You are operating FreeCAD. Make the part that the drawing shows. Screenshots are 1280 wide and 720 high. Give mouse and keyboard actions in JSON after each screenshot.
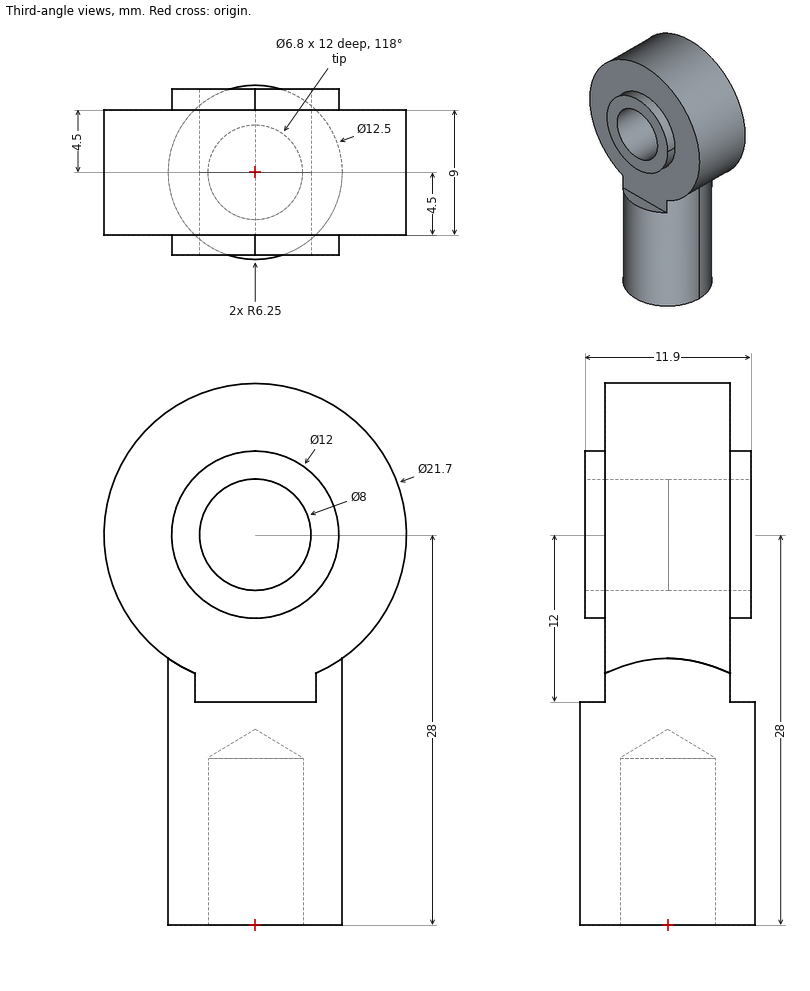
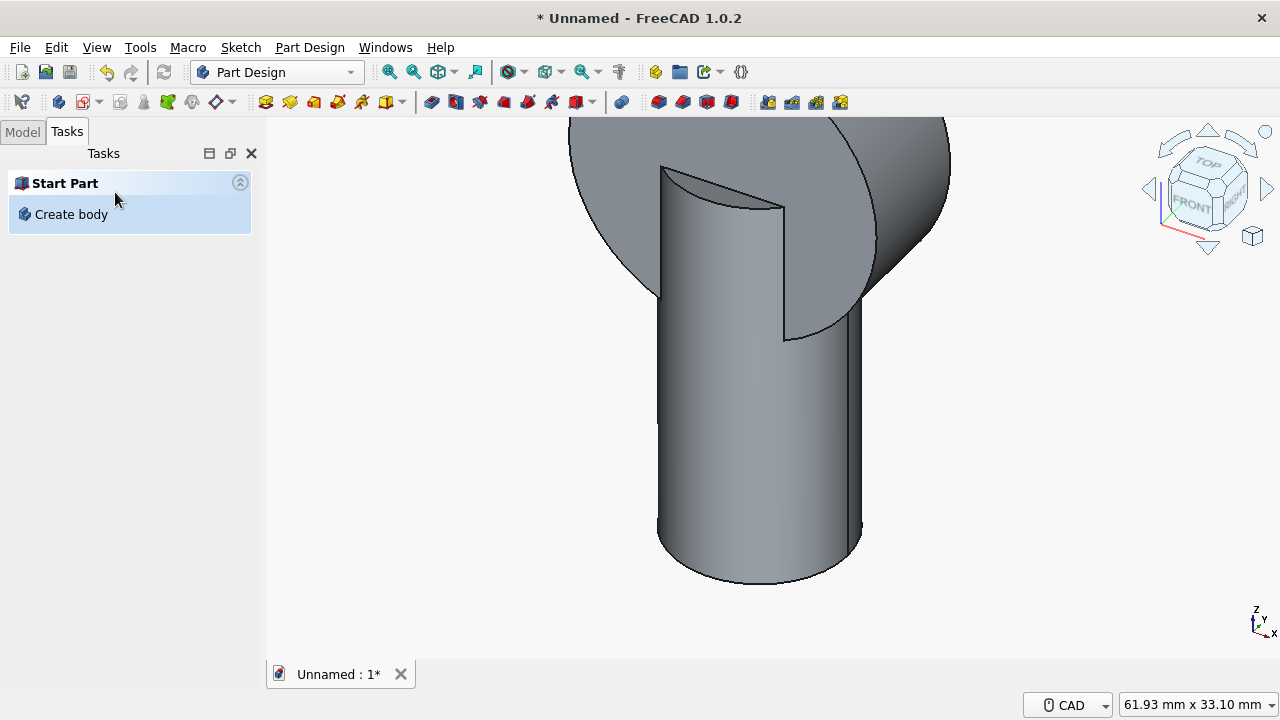
{"action": "key", "text": "v f"}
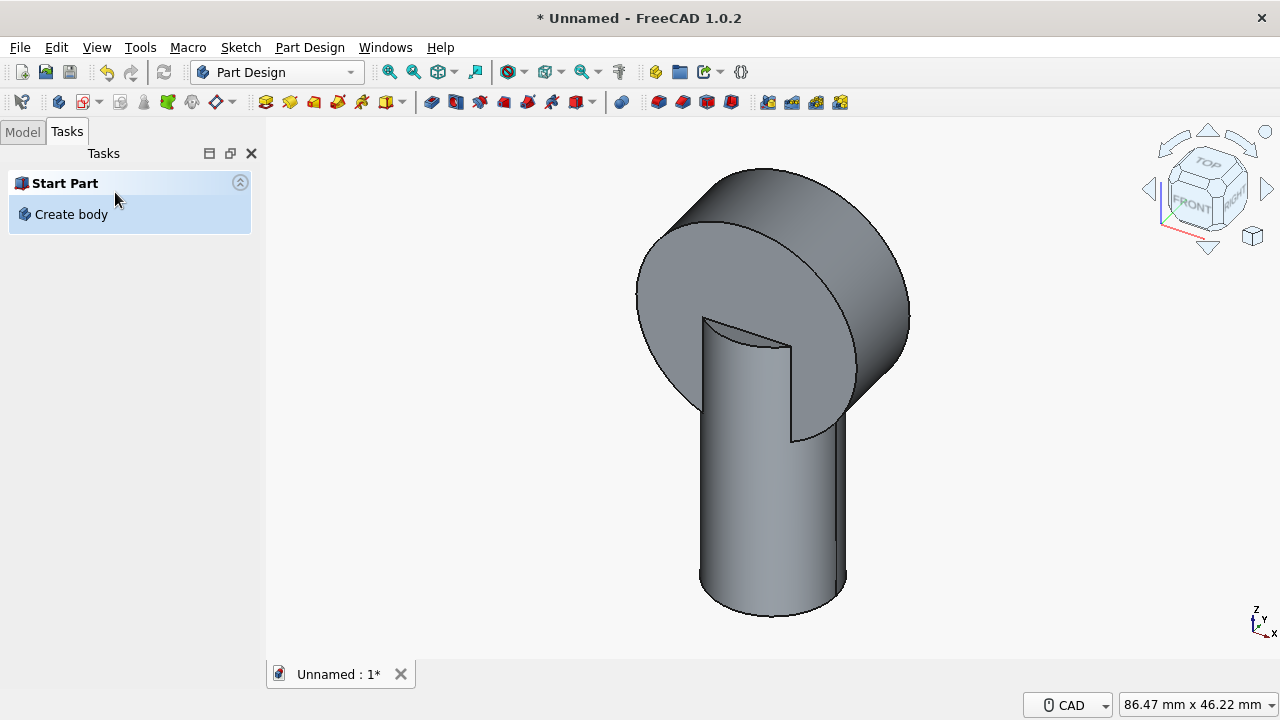
{"action": "left_click", "coordinate": [23, 131]}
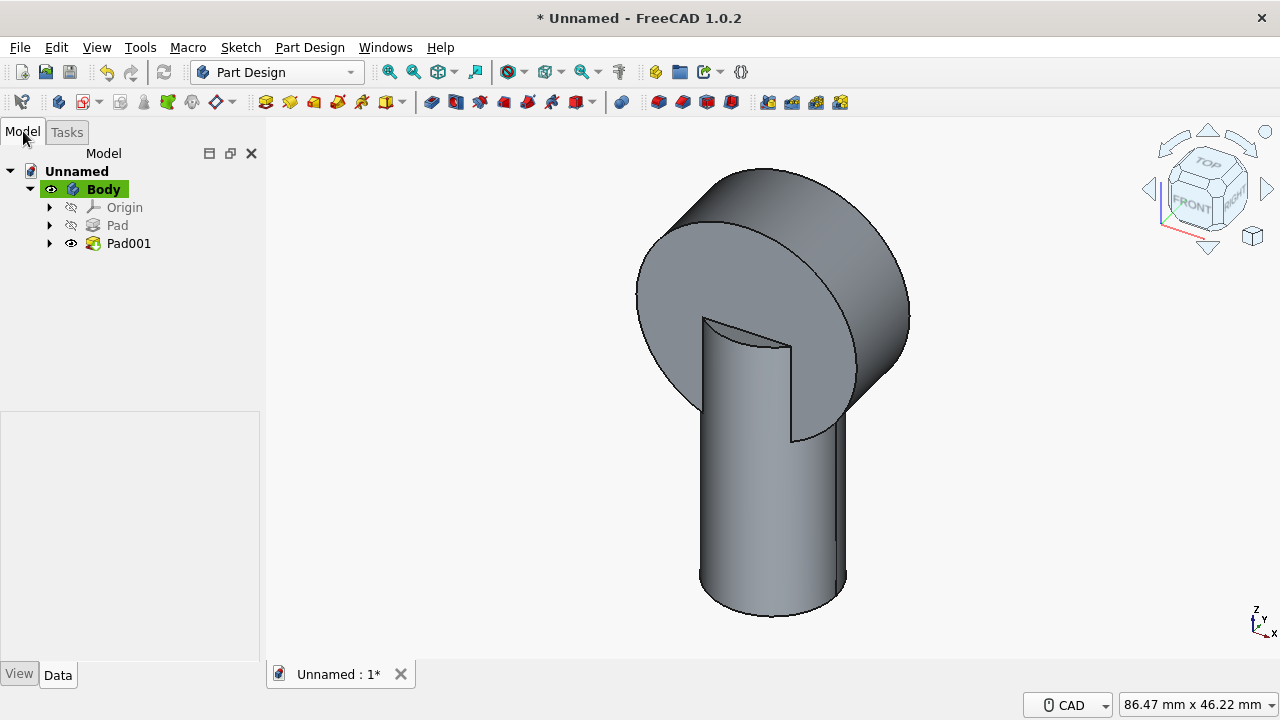
{"action": "left_click", "coordinate": [50, 207]}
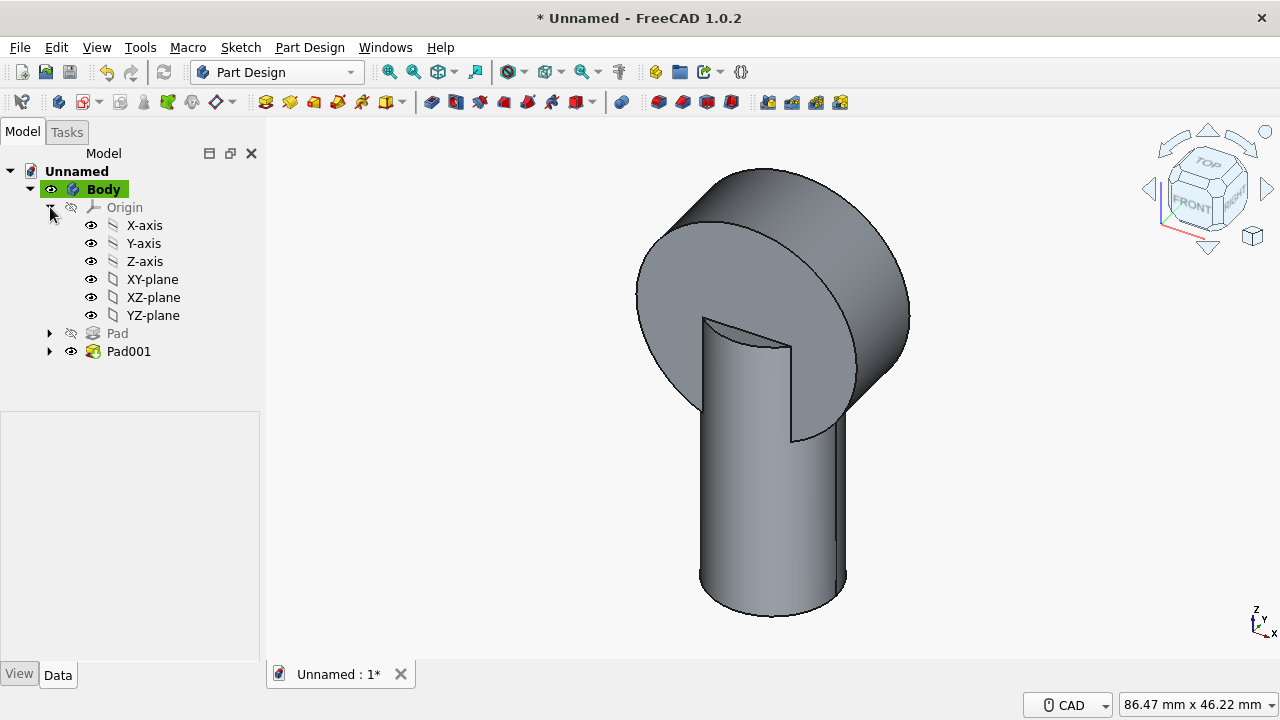
{"action": "left_click", "coordinate": [136, 279]}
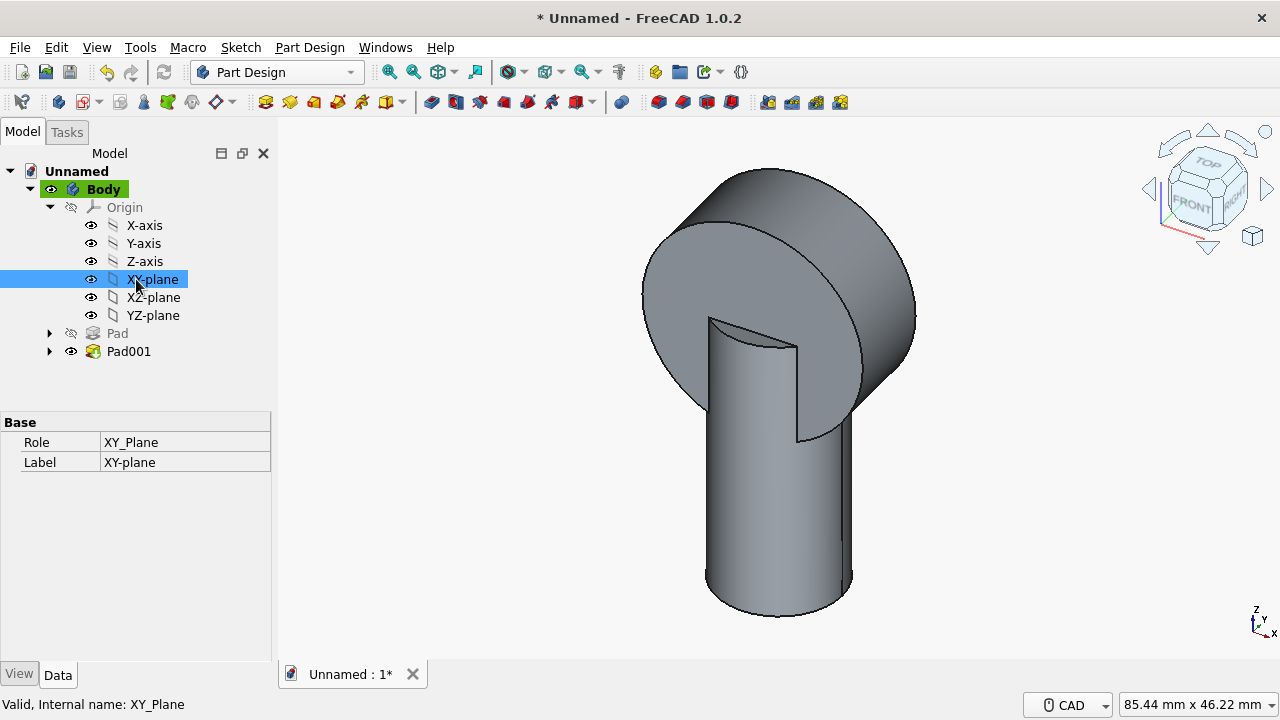
{"action": "left_click", "coordinate": [216, 102]}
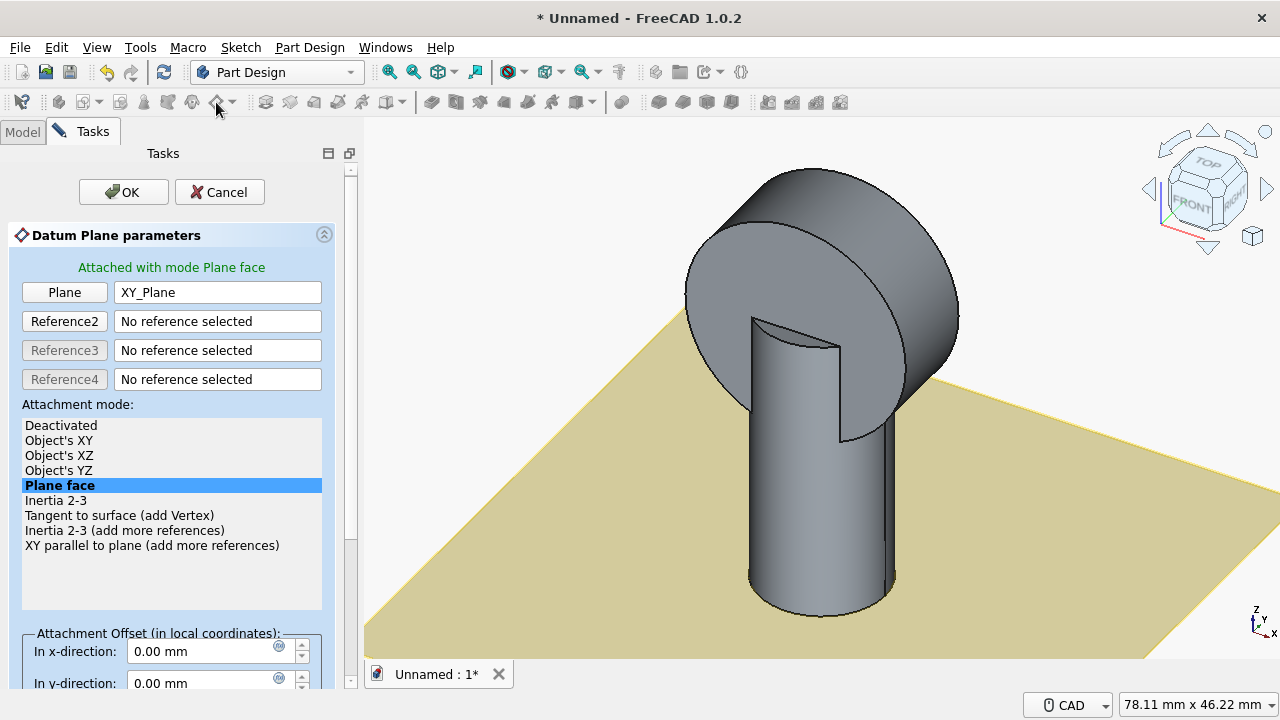
{"action": "scroll", "coordinate": [351, 426], "scroll_direction": "down", "scroll_amount": 2}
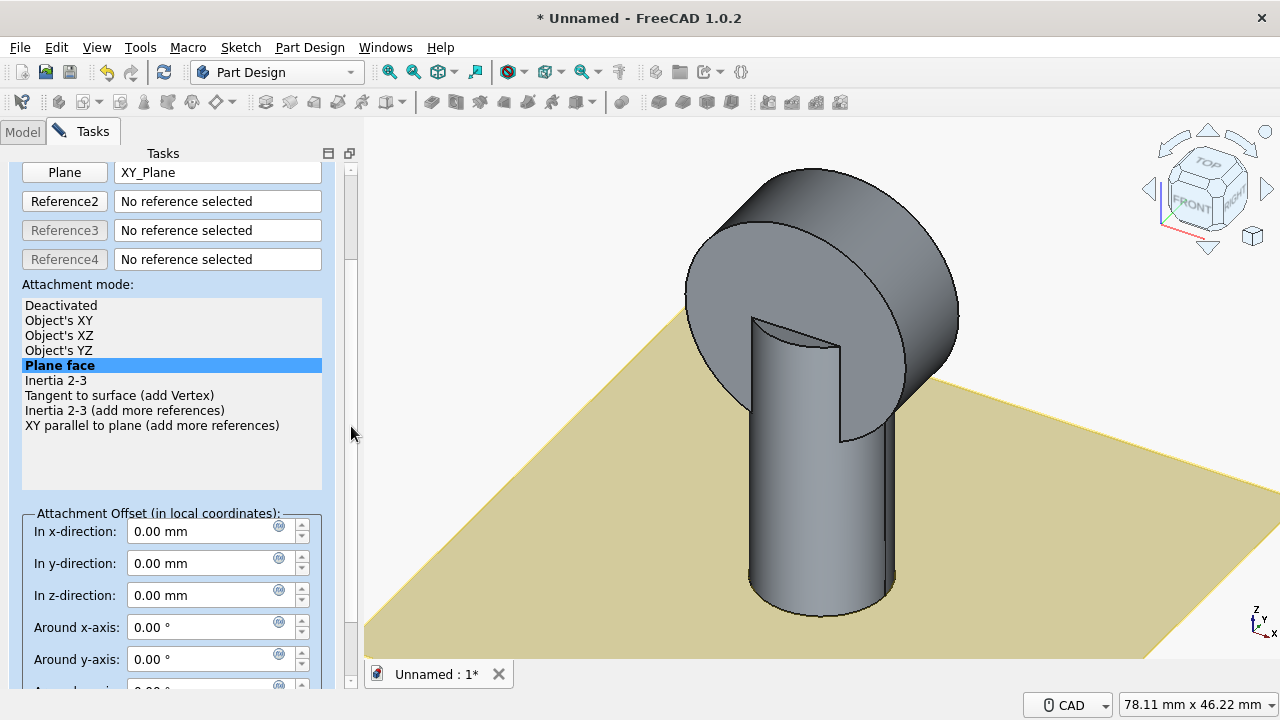
{"action": "triple_click", "coordinate": [210, 595]}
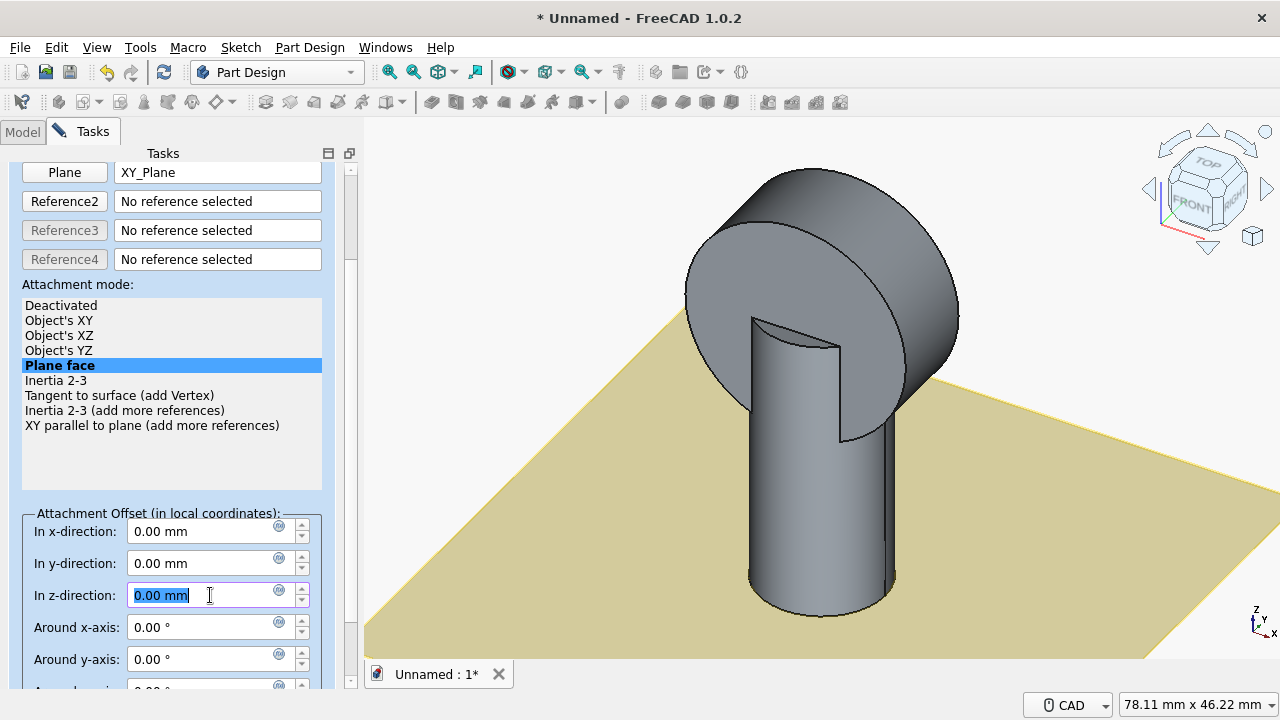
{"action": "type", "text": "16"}
{"action": "key", "text": "Tab"}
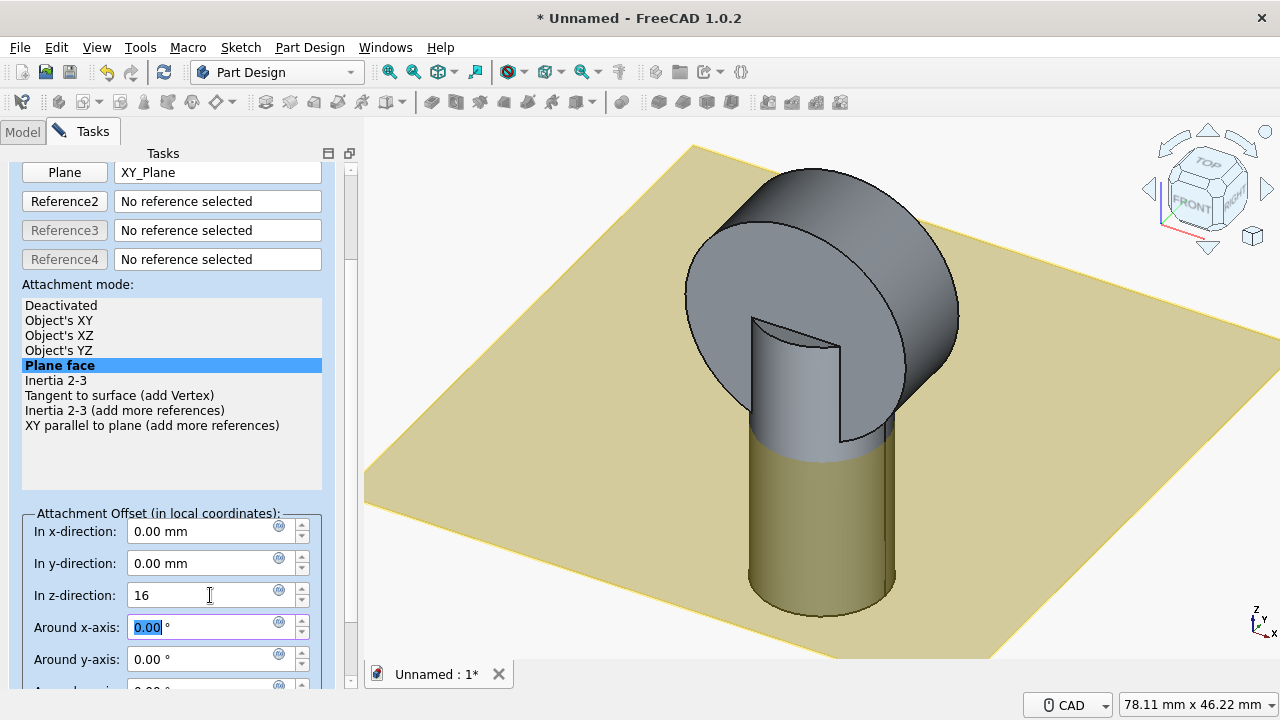
{"action": "scroll", "coordinate": [351, 426], "scroll_direction": "up", "scroll_amount": 3}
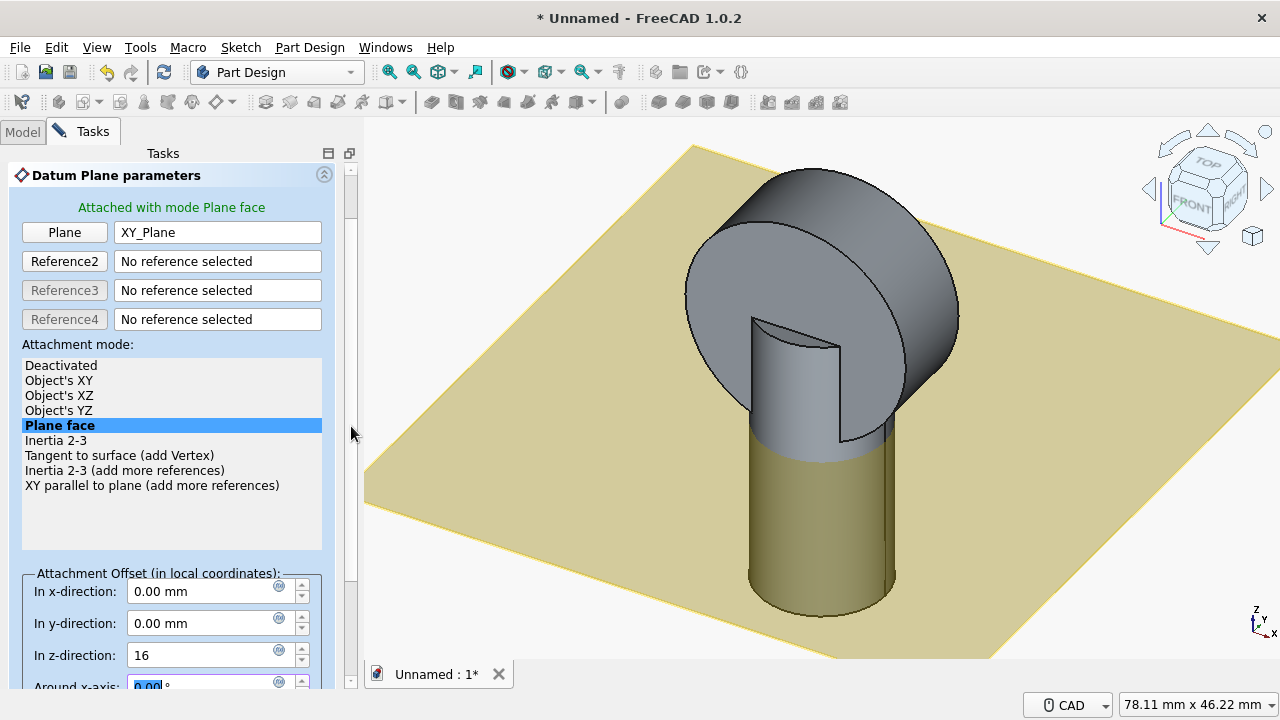
{"action": "left_click", "coordinate": [124, 192]}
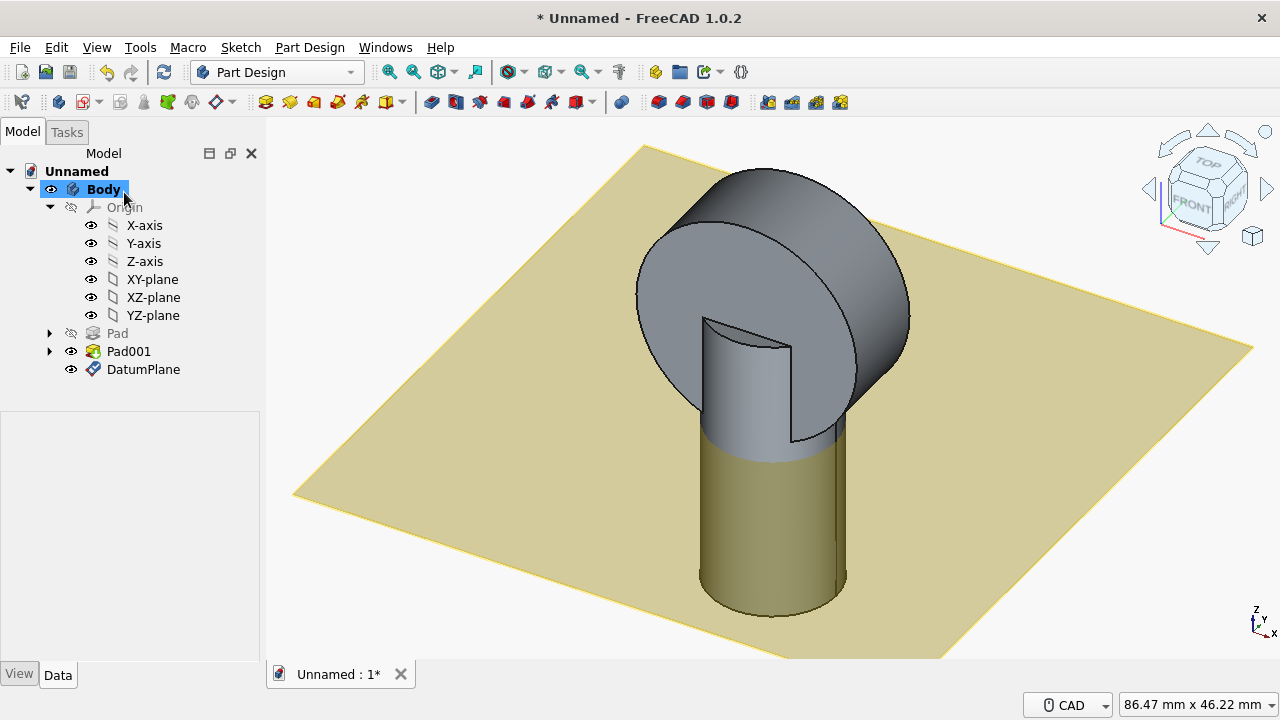
{"action": "left_click", "coordinate": [116, 369]}